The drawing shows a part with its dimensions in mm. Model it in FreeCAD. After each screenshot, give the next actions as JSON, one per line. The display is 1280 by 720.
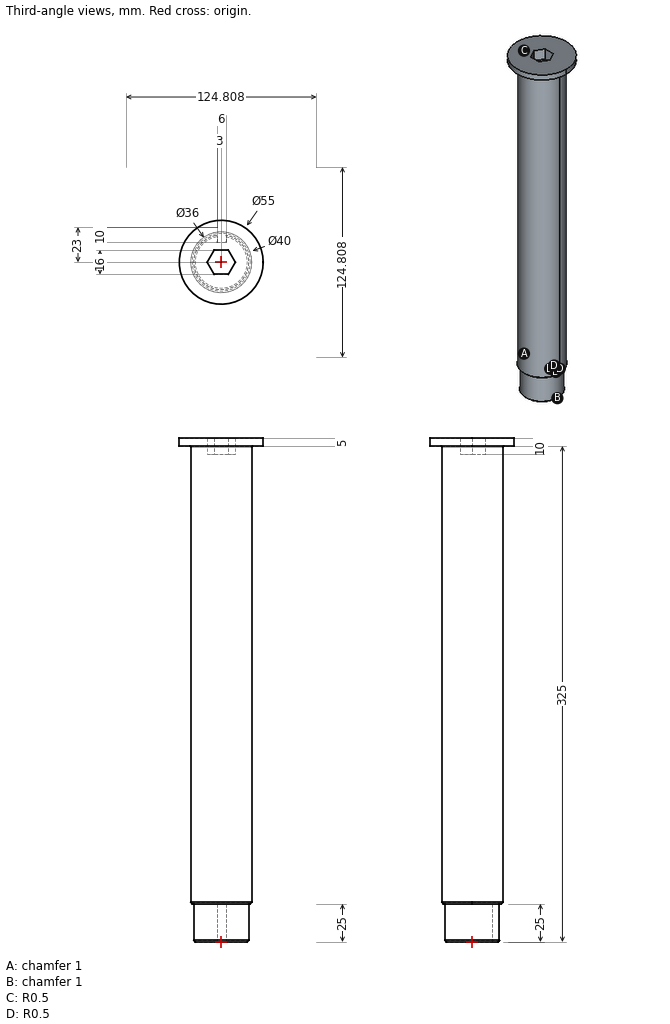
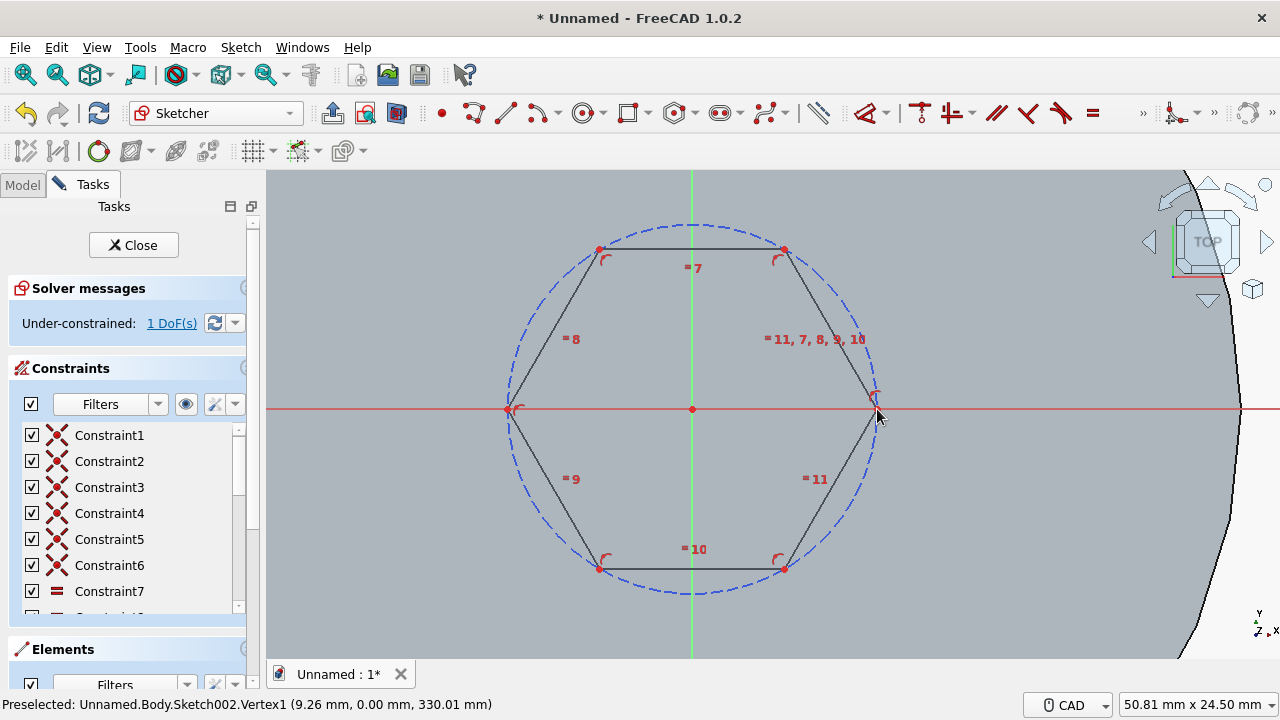
{"action": "left_click", "coordinate": [866, 114]}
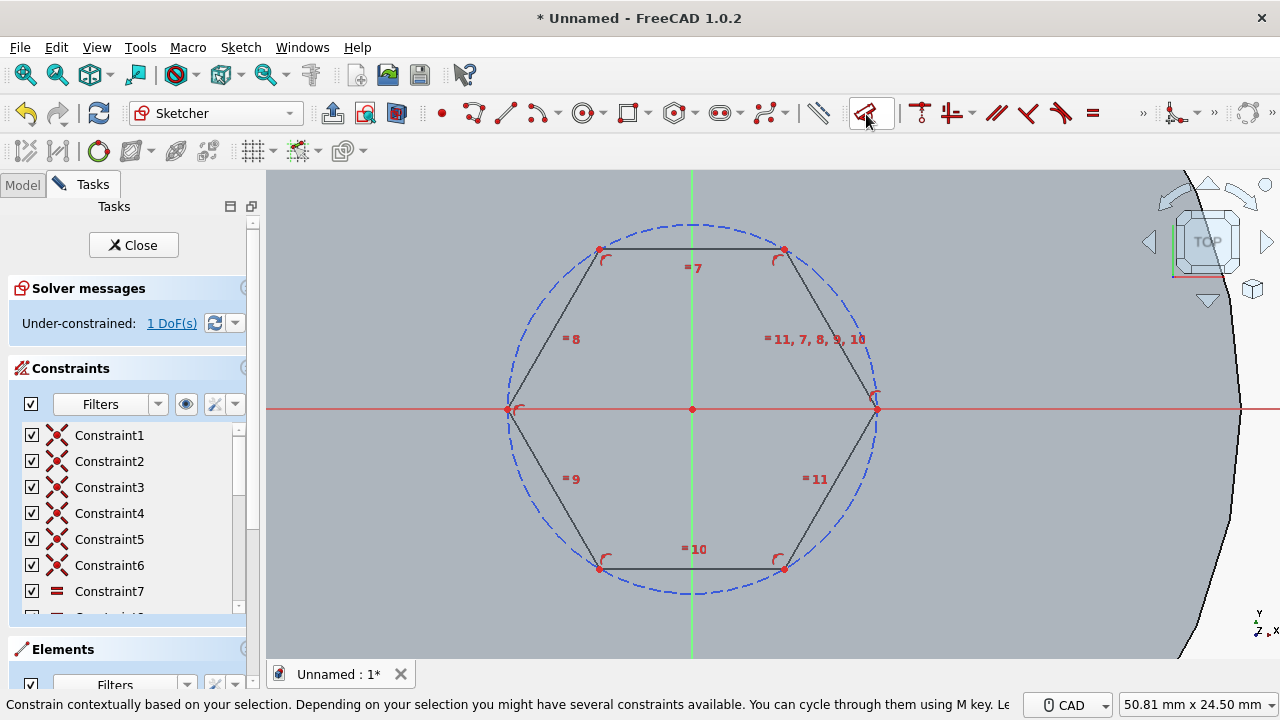
{"action": "left_click", "coordinate": [600, 569]}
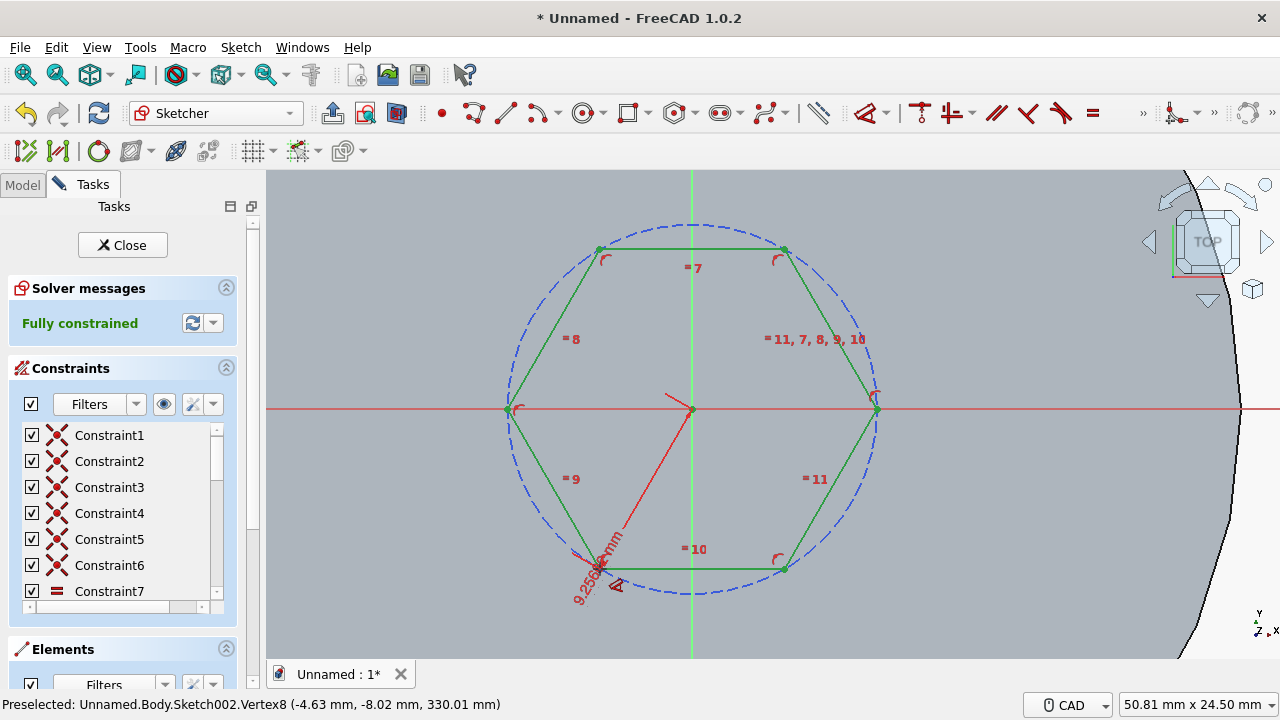
{"action": "left_click", "coordinate": [785, 249]}
{"action": "left_click", "coordinate": [566, 336]}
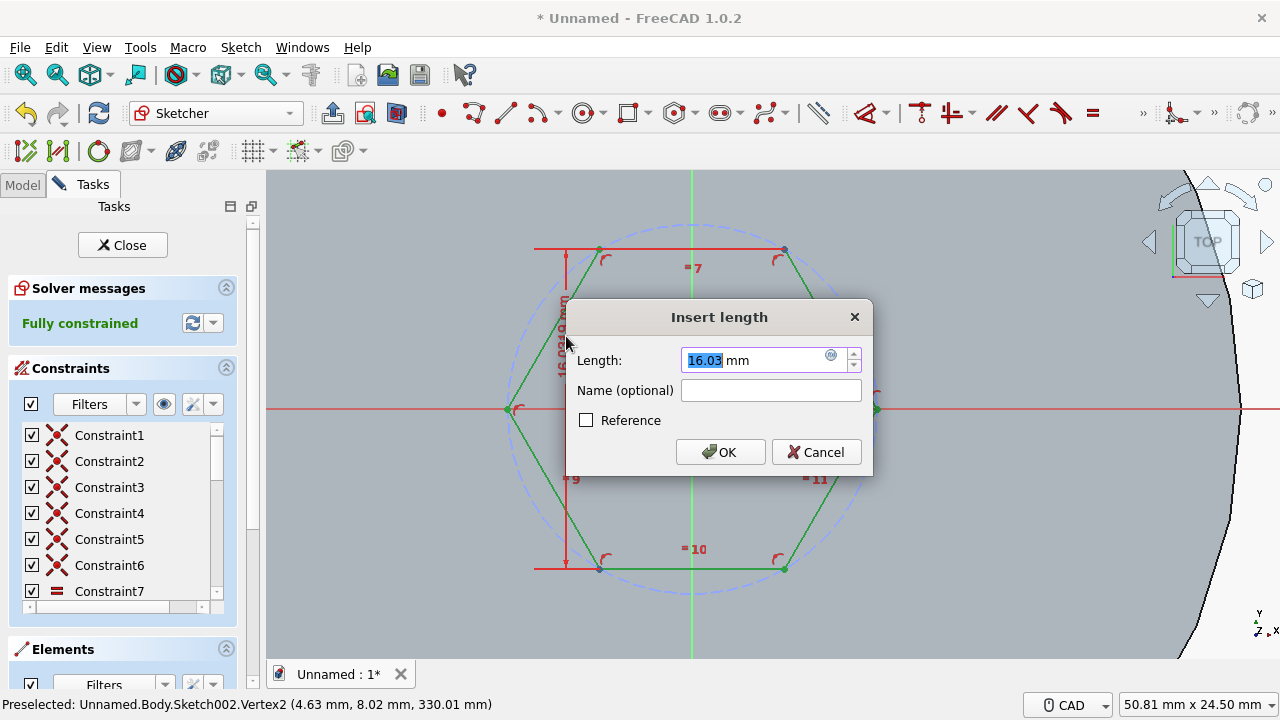
{"action": "type", "text": "16"}
{"action": "key", "text": "Return"}
{"action": "key", "text": "Escape"}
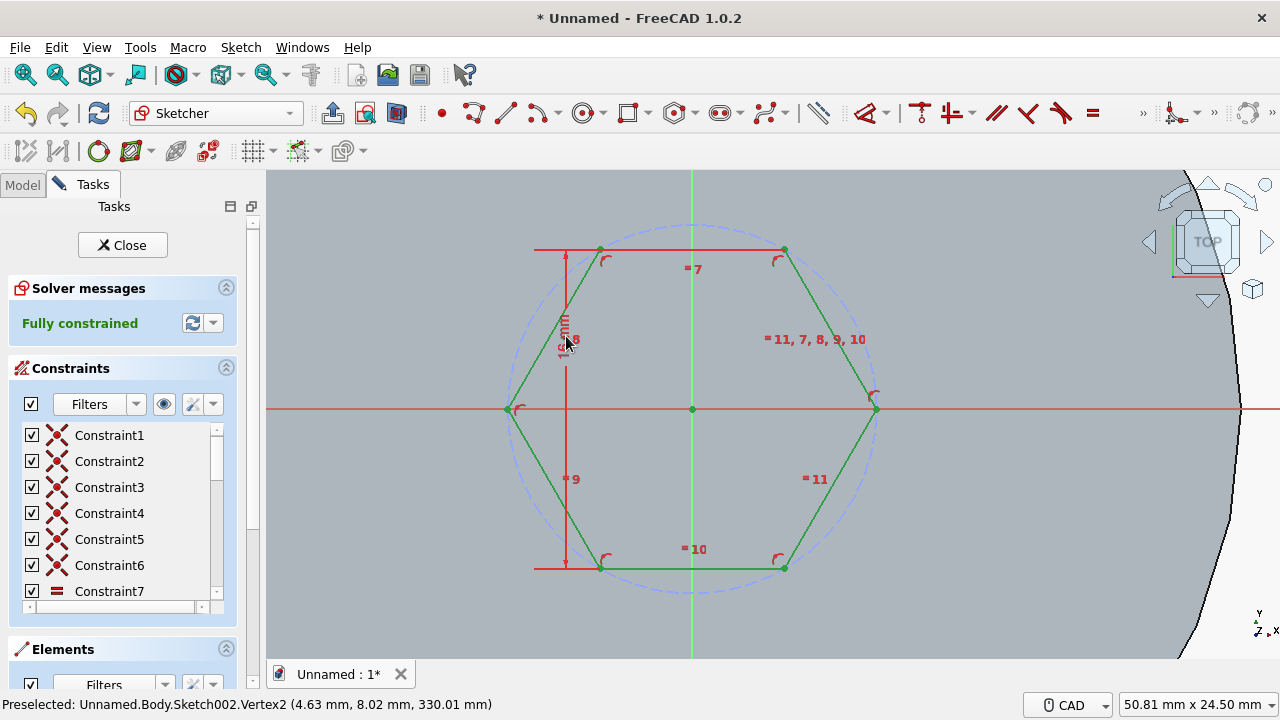
{"action": "left_click", "coordinate": [123, 245]}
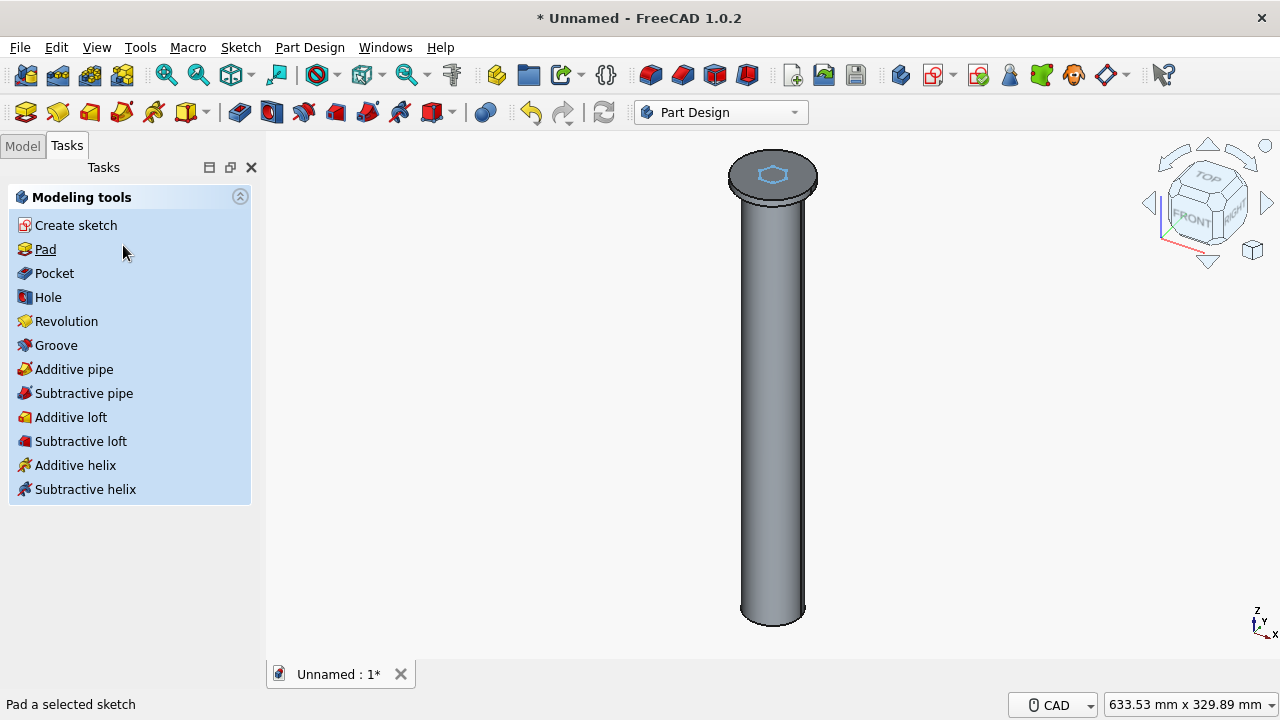
{"action": "left_click", "coordinate": [240, 112]}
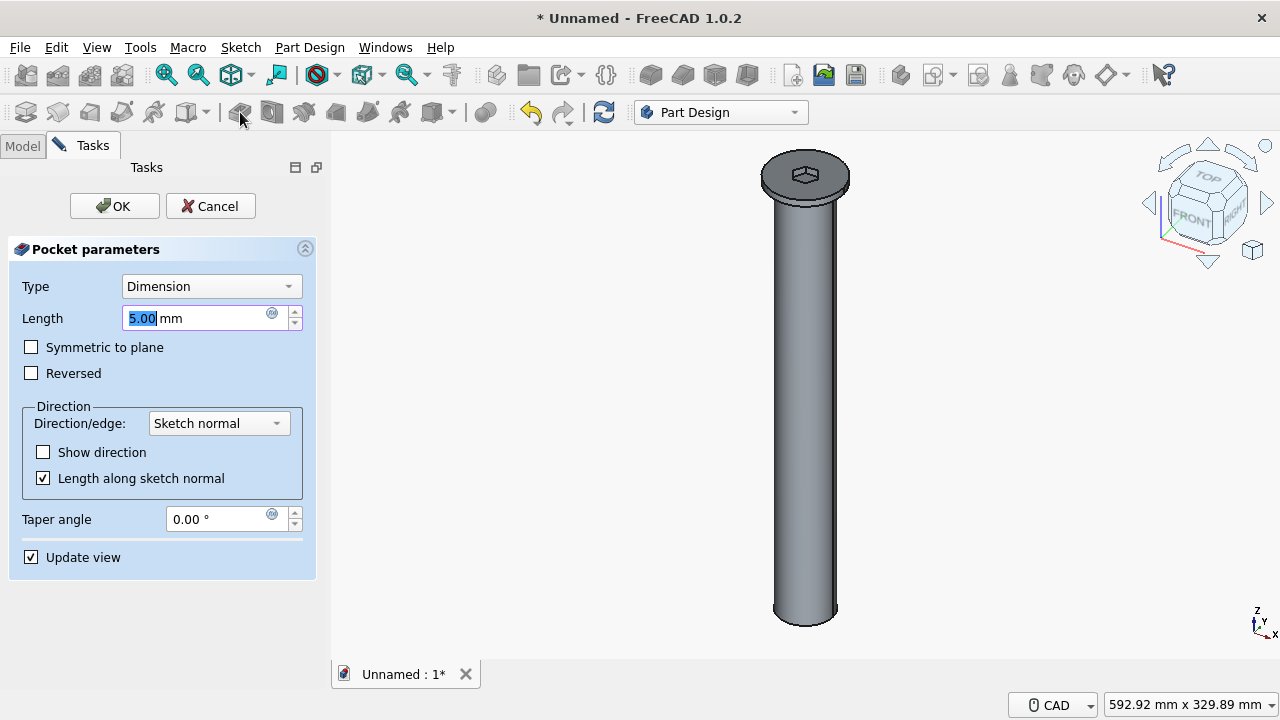
{"action": "type", "text": "10"}
{"action": "key", "text": "Tab"}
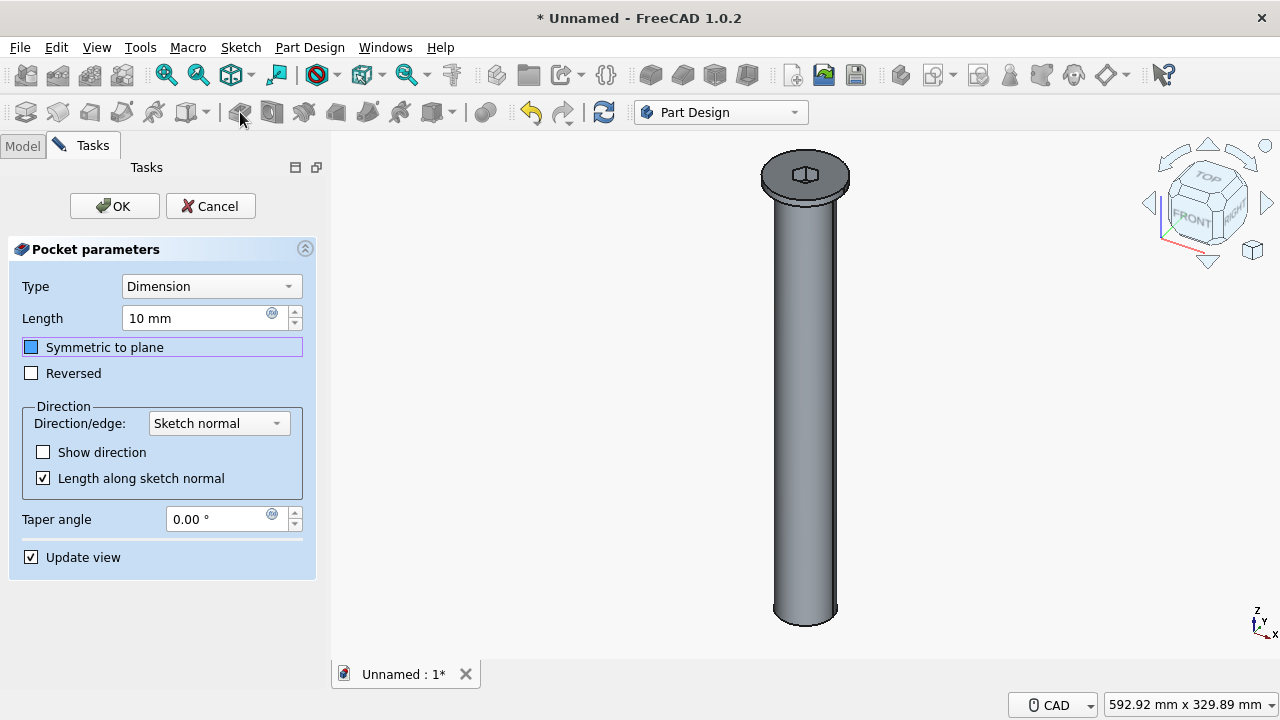
{"action": "left_click", "coordinate": [115, 206]}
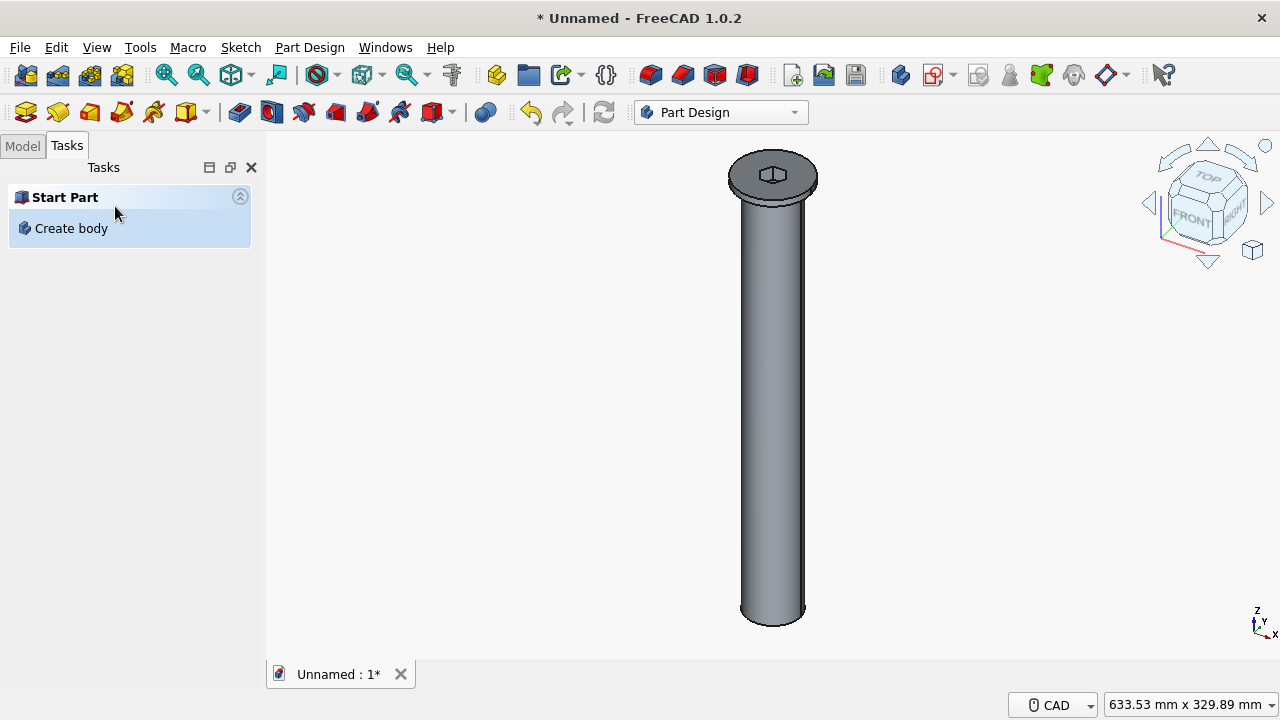
{"action": "key", "text": "5"}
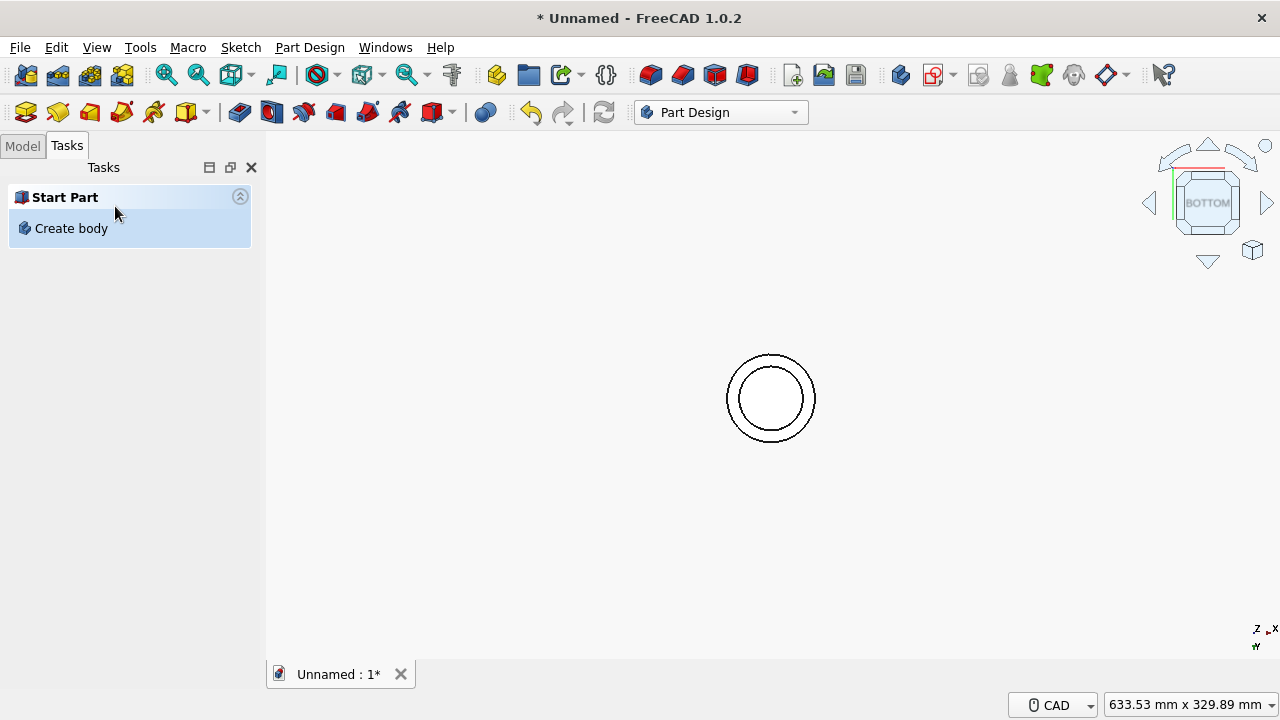
{"action": "left_click", "coordinate": [168, 76]}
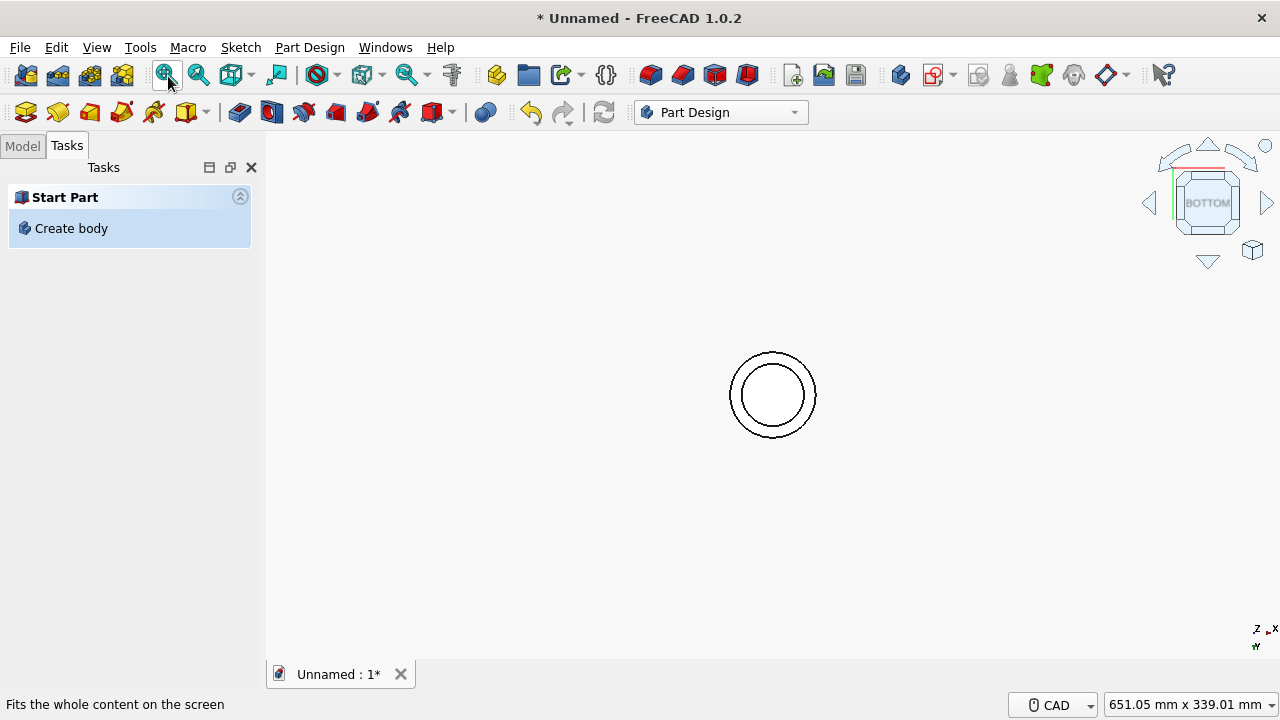
{"action": "left_click", "coordinate": [773, 394]}